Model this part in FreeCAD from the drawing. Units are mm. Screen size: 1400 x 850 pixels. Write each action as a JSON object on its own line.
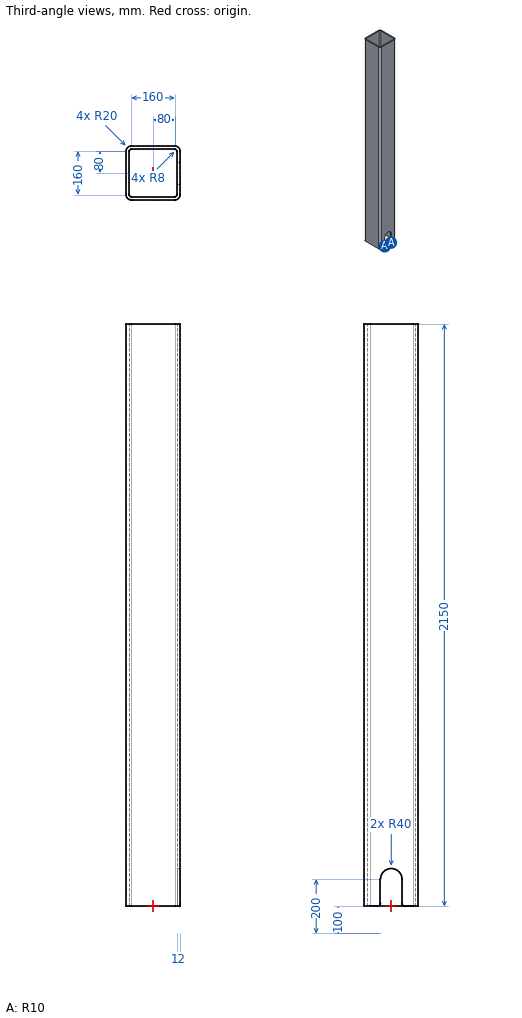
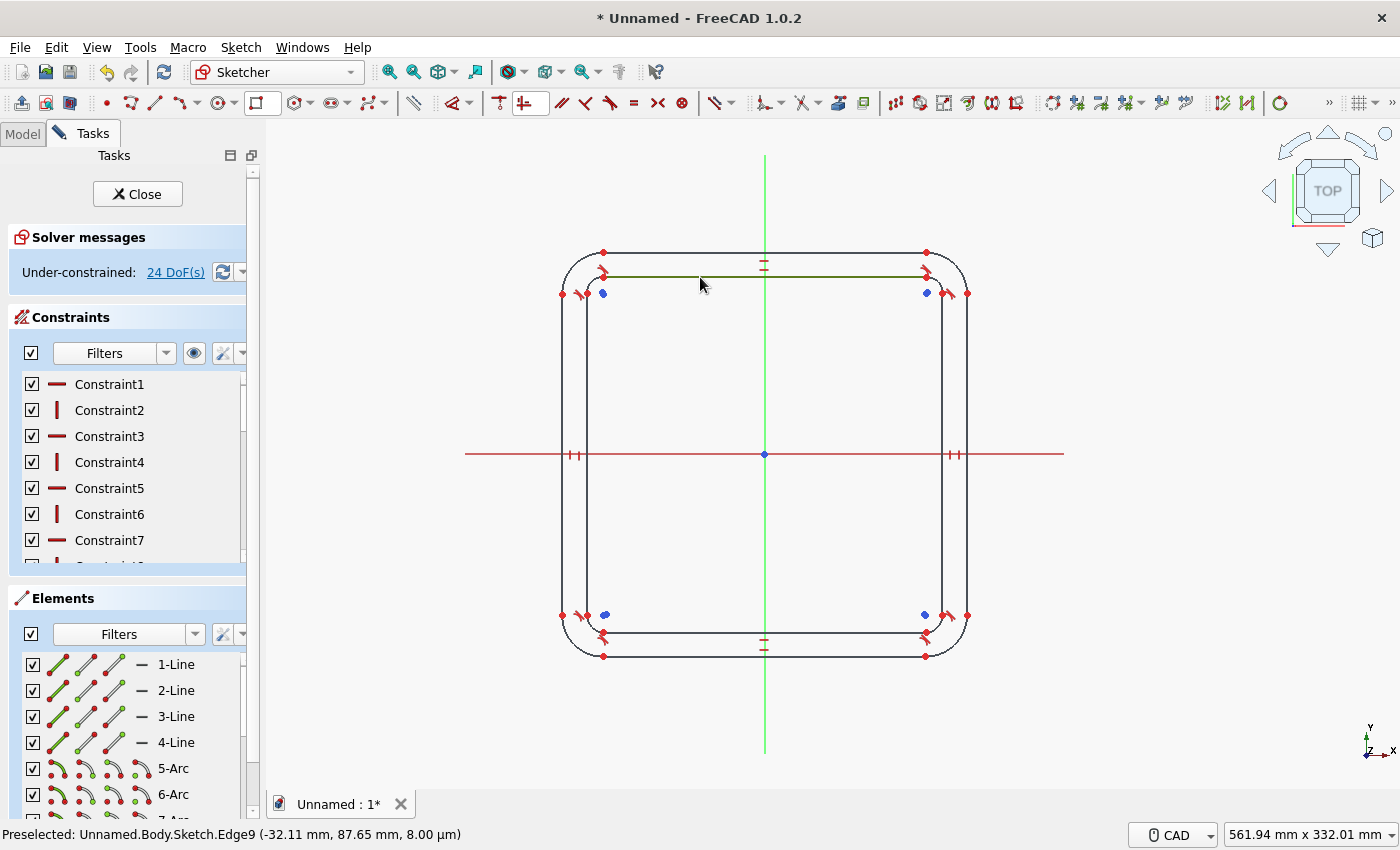
{"action": "left_click", "coordinate": [938, 282]}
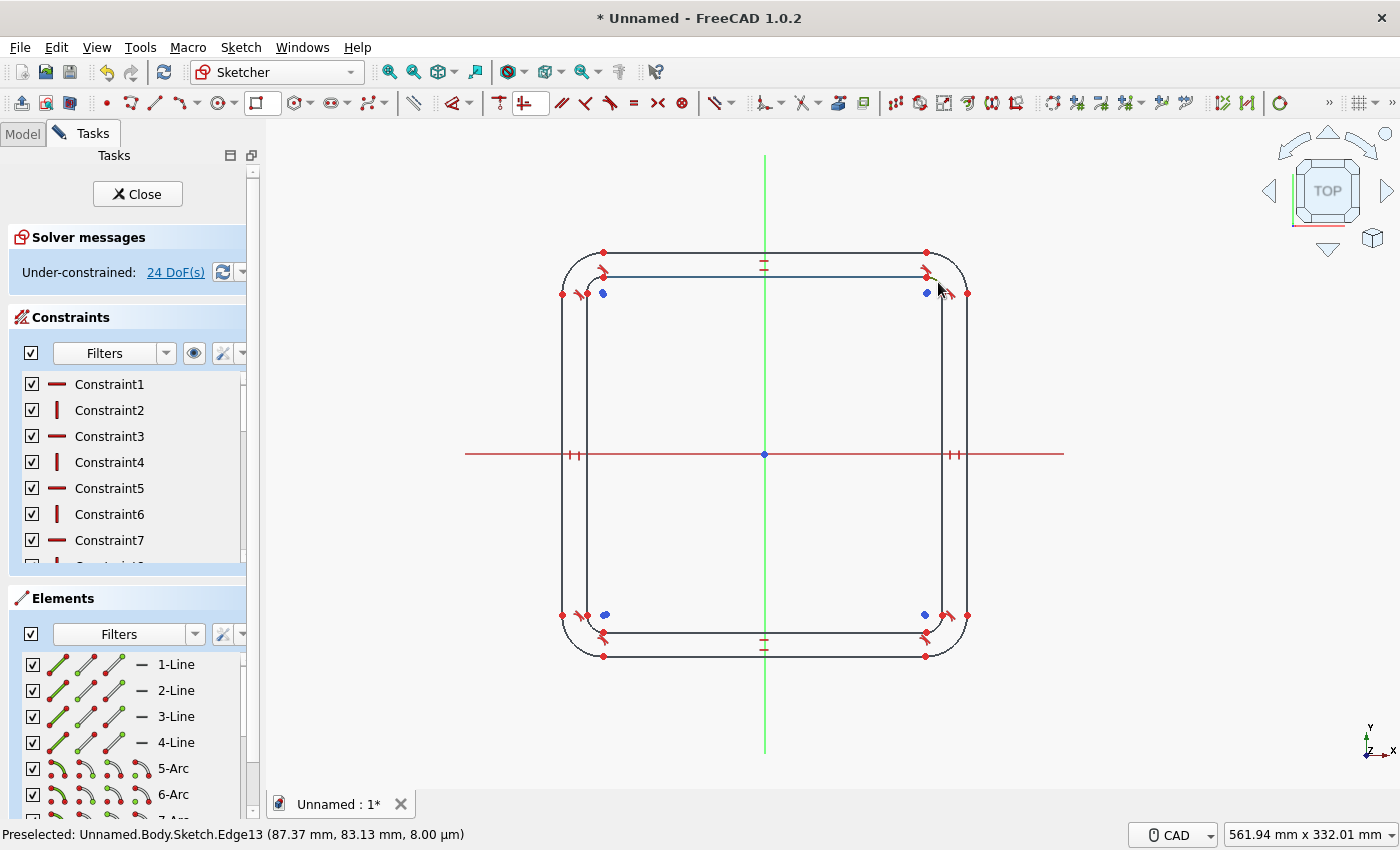
{"action": "left_click", "coordinate": [610, 104]}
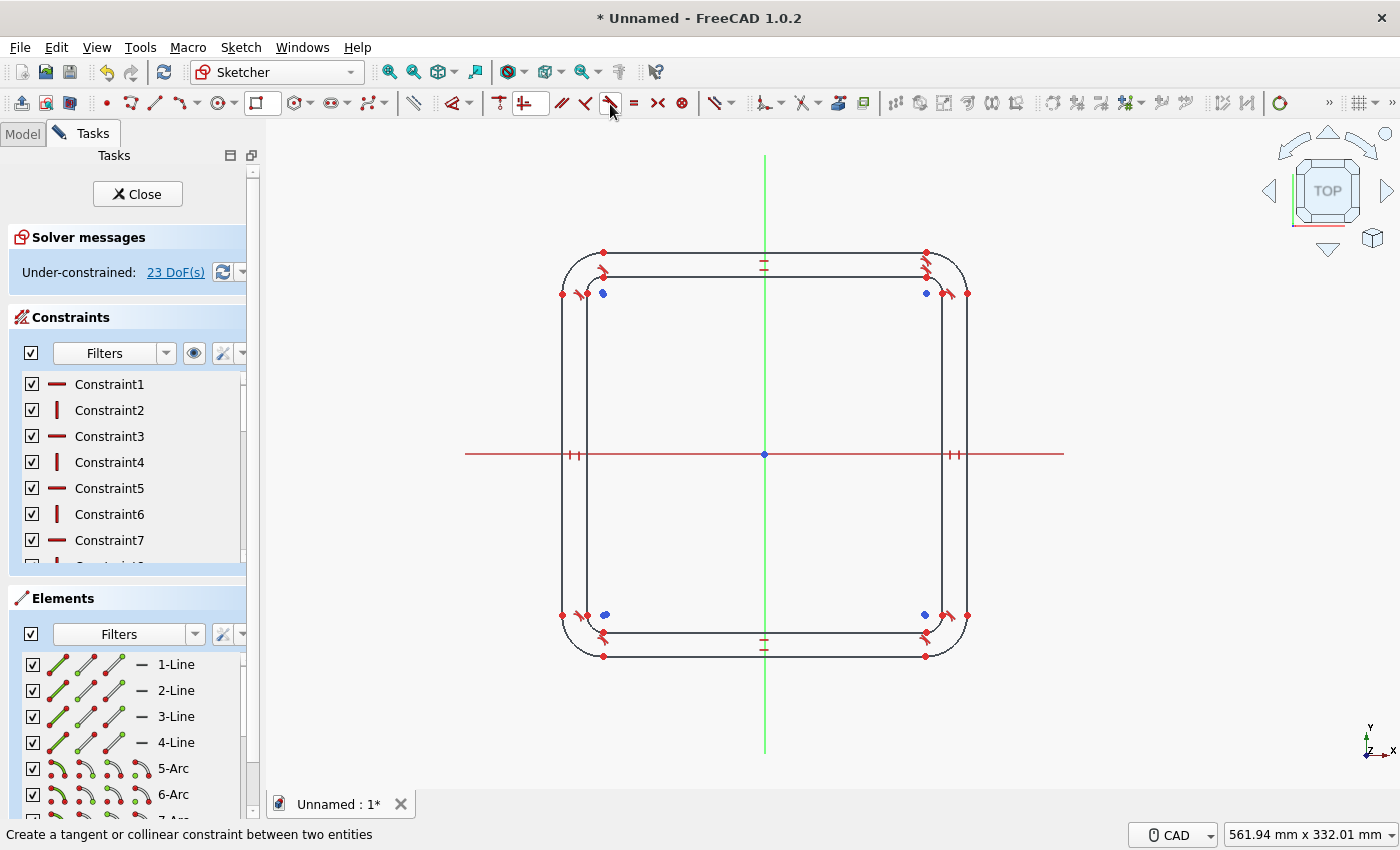
{"action": "left_click", "coordinate": [700, 277]}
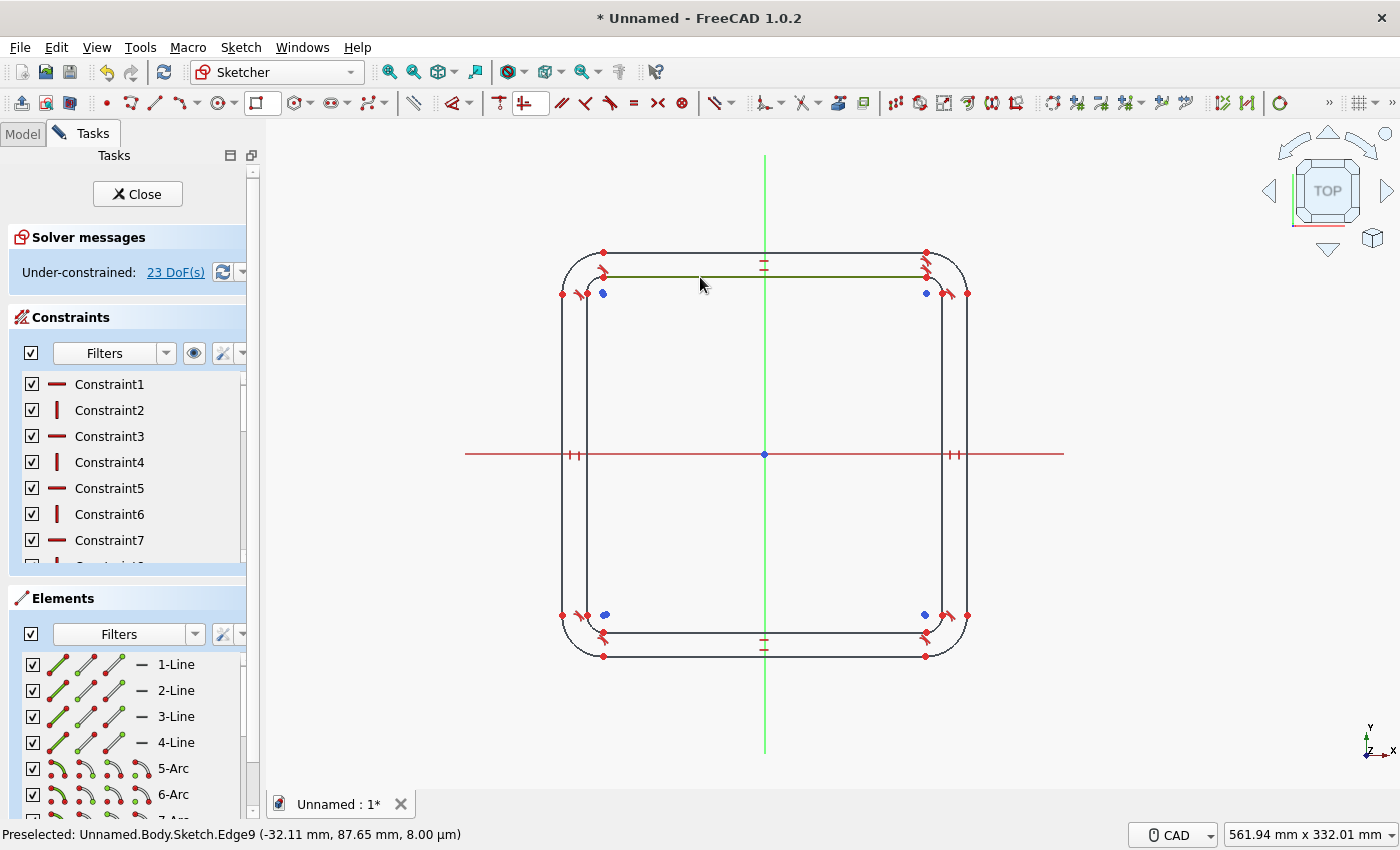
{"action": "left_click", "coordinate": [591, 282]}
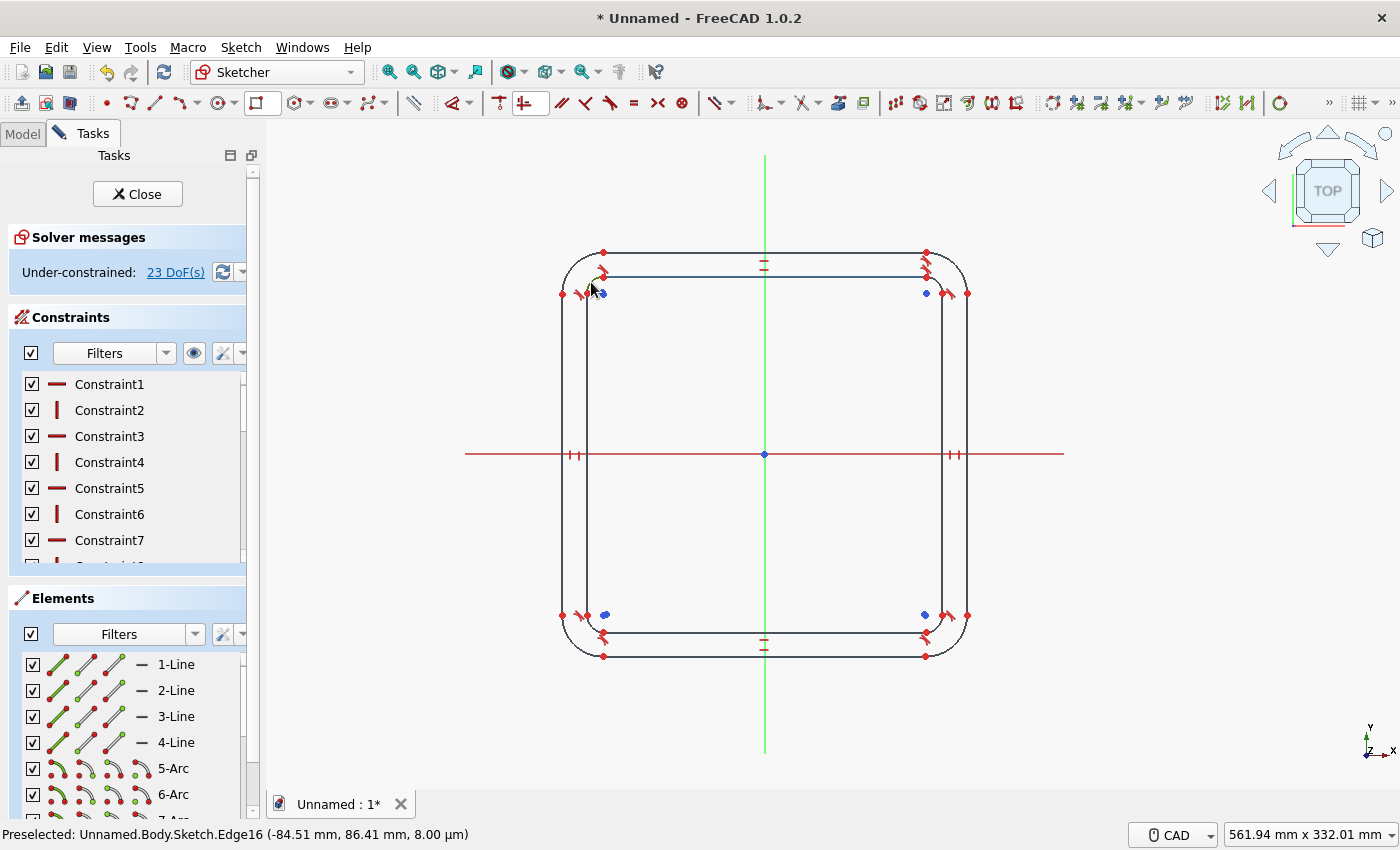
{"action": "left_click", "coordinate": [610, 104]}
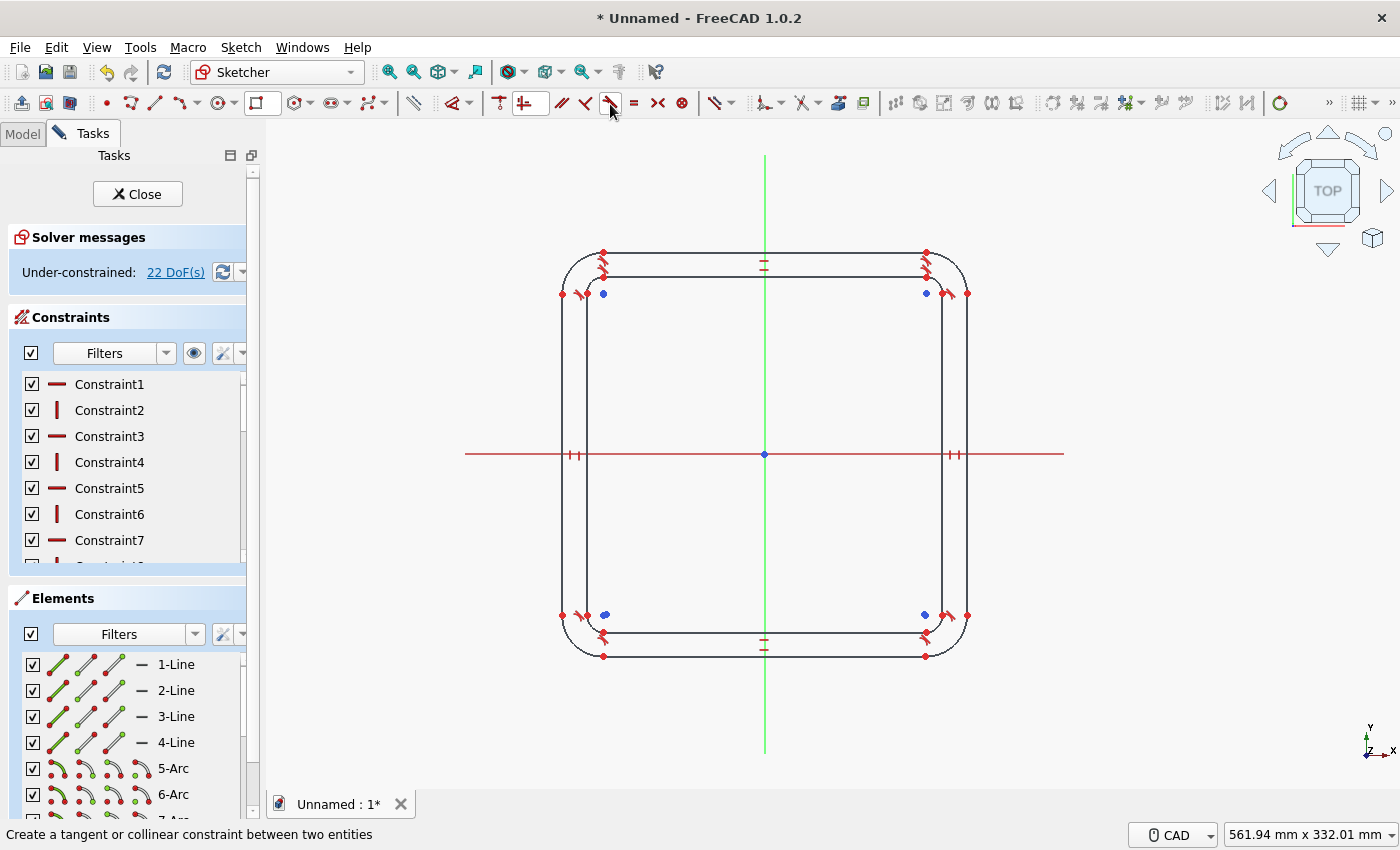
{"action": "left_click", "coordinate": [942, 390]}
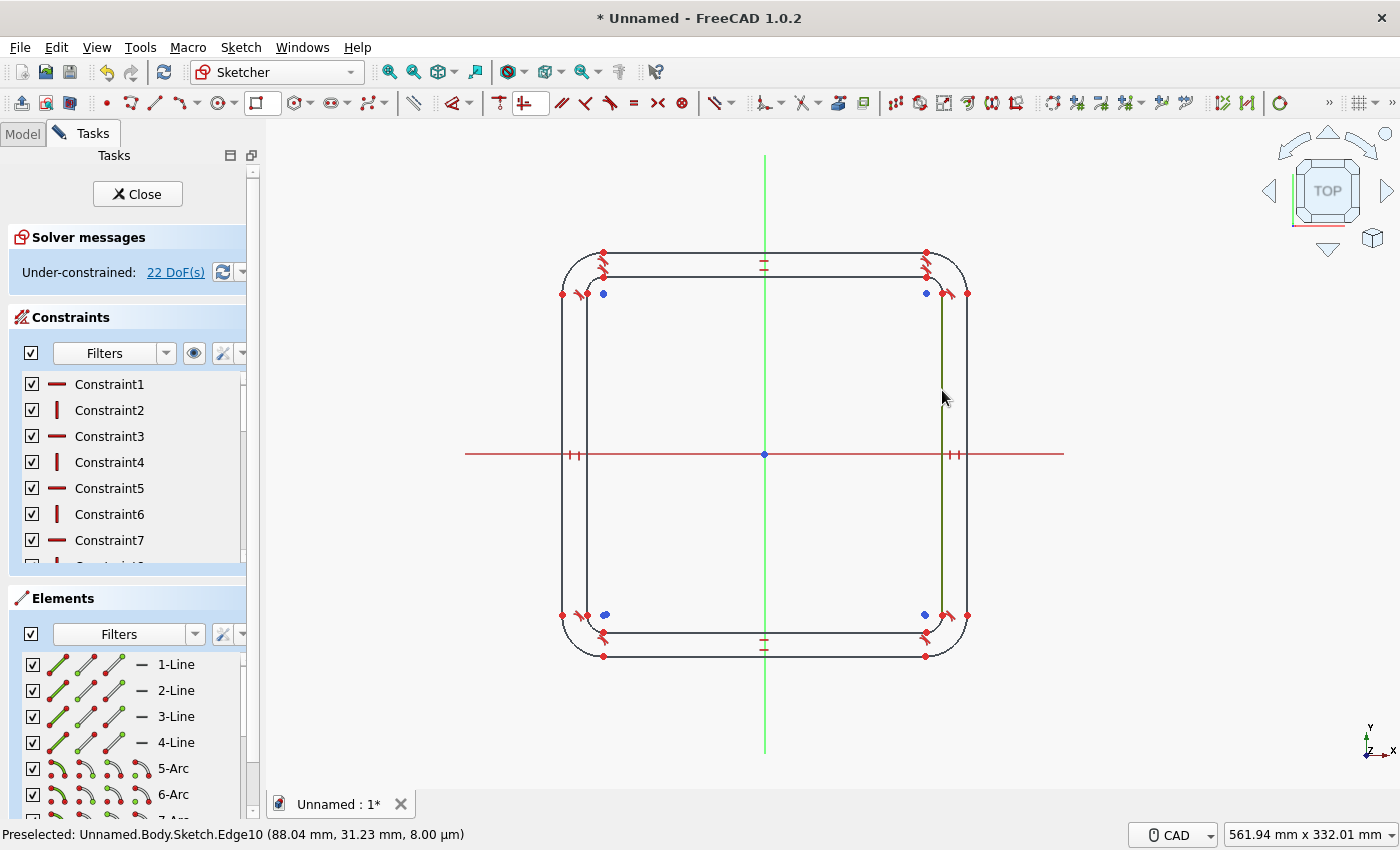
{"action": "left_click", "coordinate": [938, 282]}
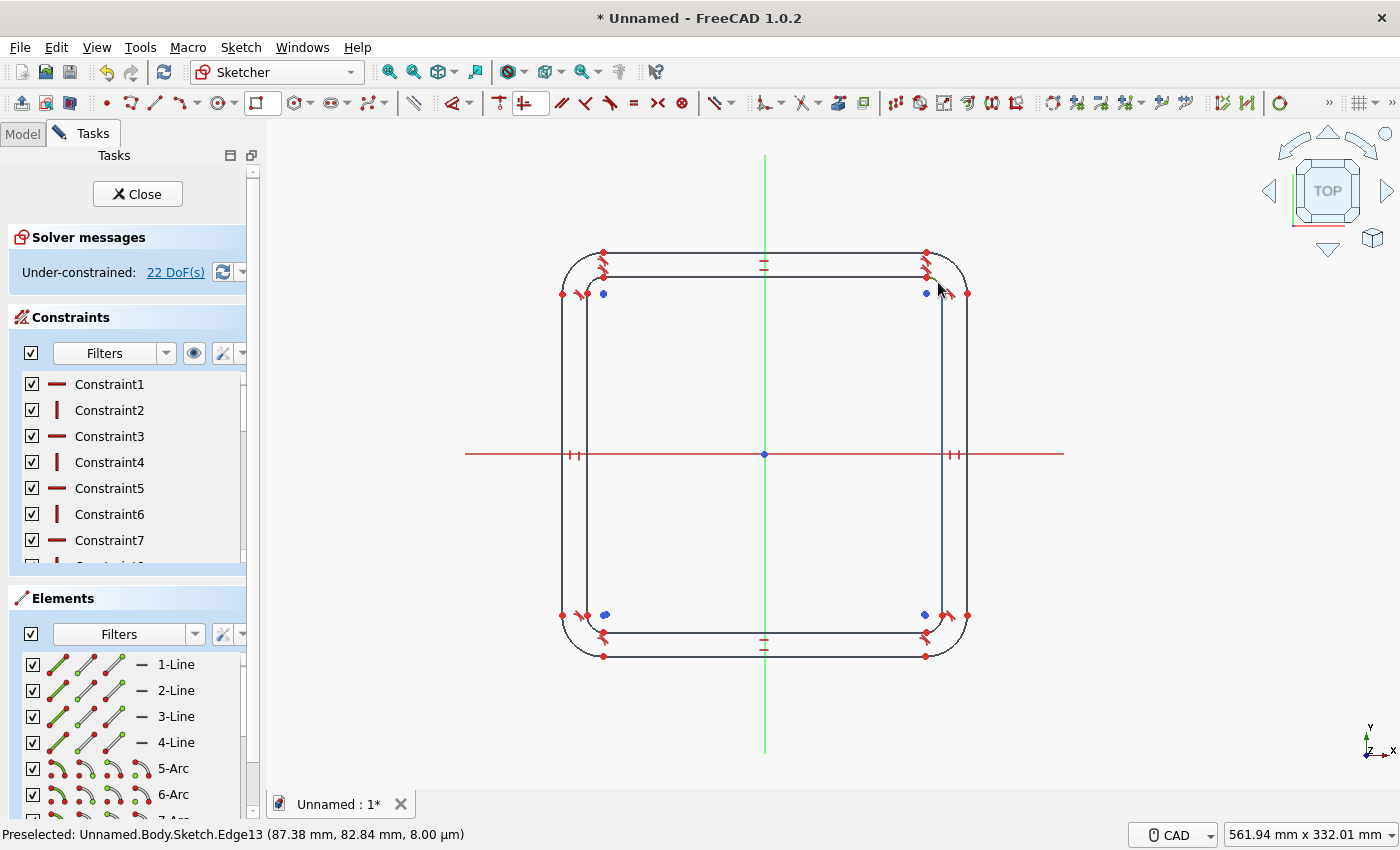
{"action": "left_click", "coordinate": [610, 104]}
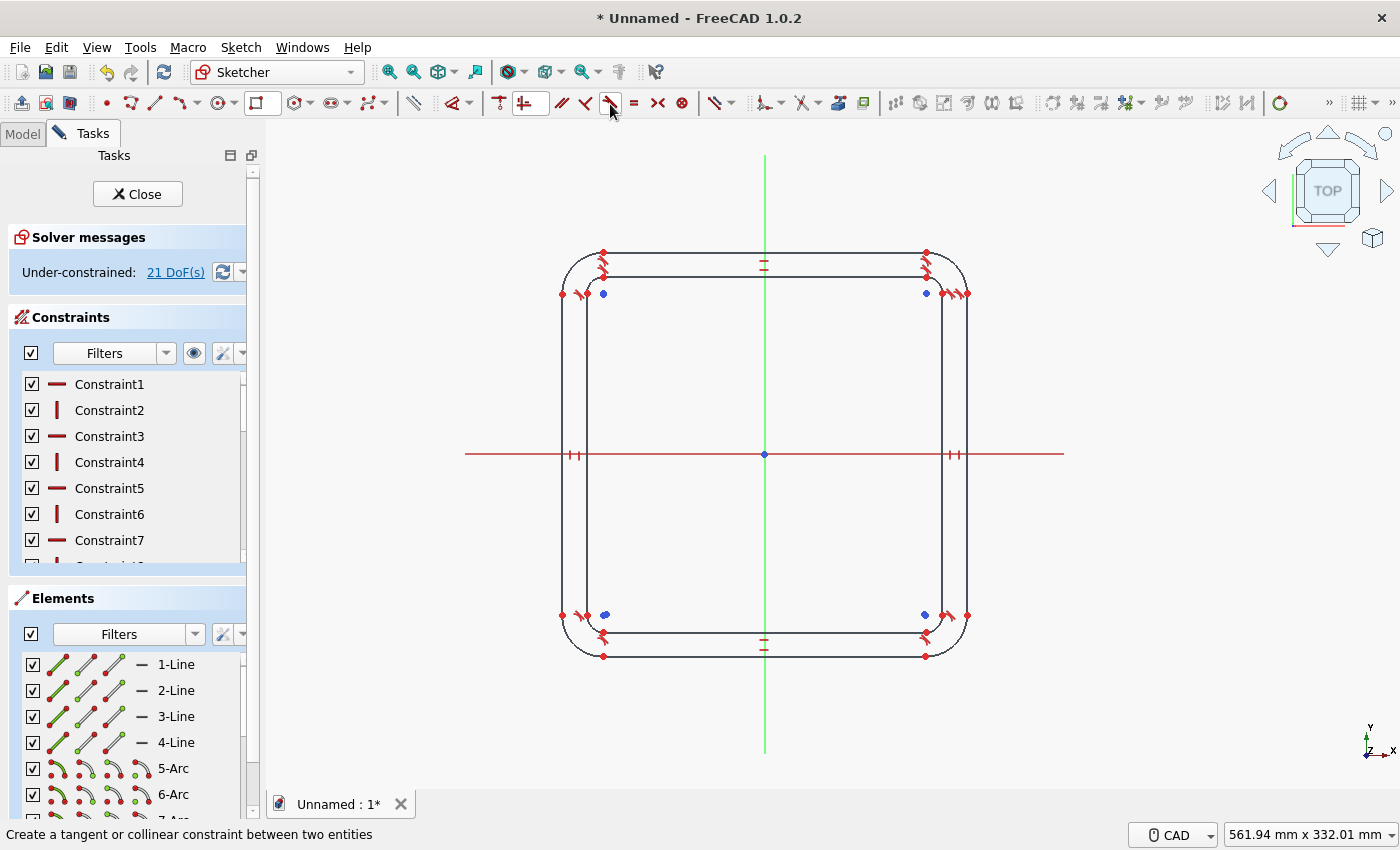
{"action": "left_click", "coordinate": [942, 390]}